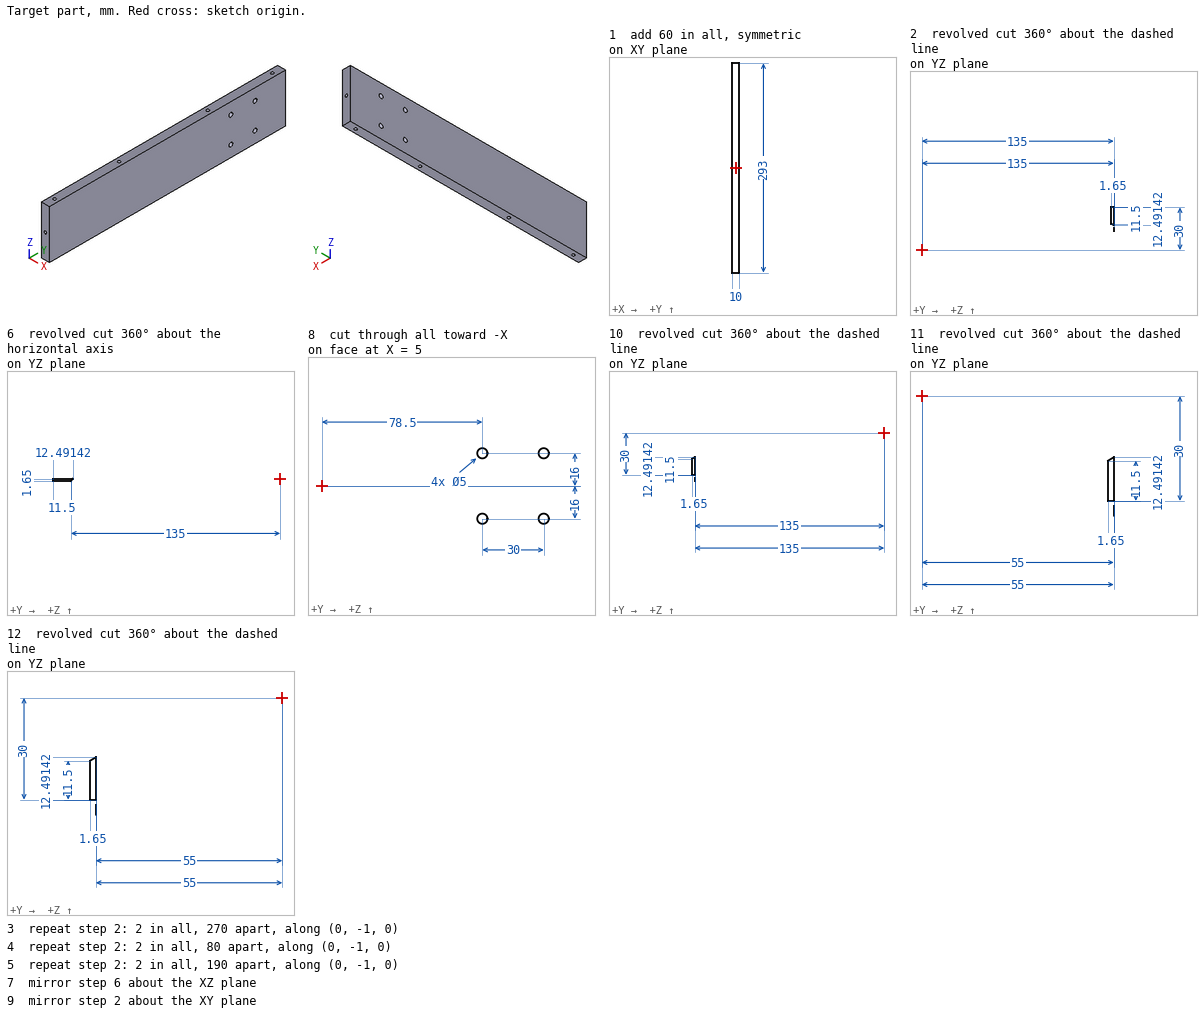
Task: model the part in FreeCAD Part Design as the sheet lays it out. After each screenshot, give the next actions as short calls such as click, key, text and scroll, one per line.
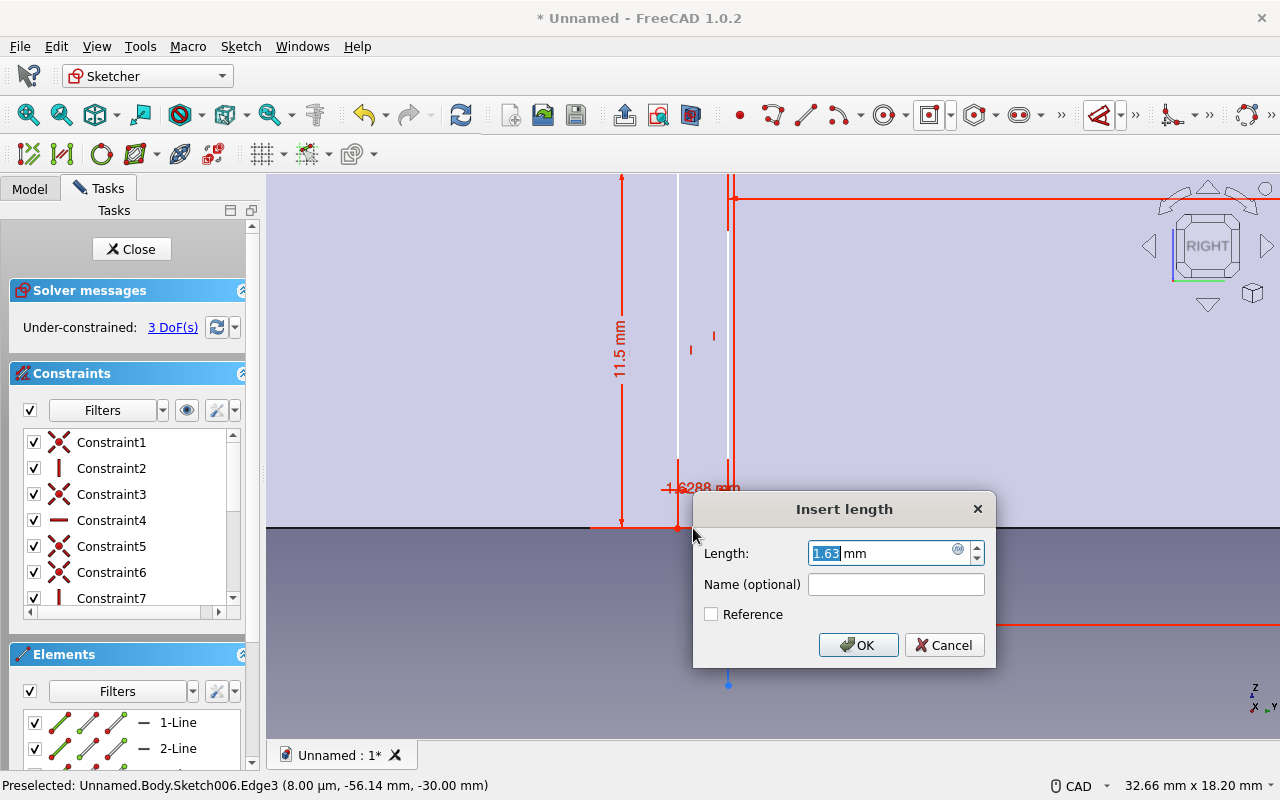
text(1.65)
key(Return)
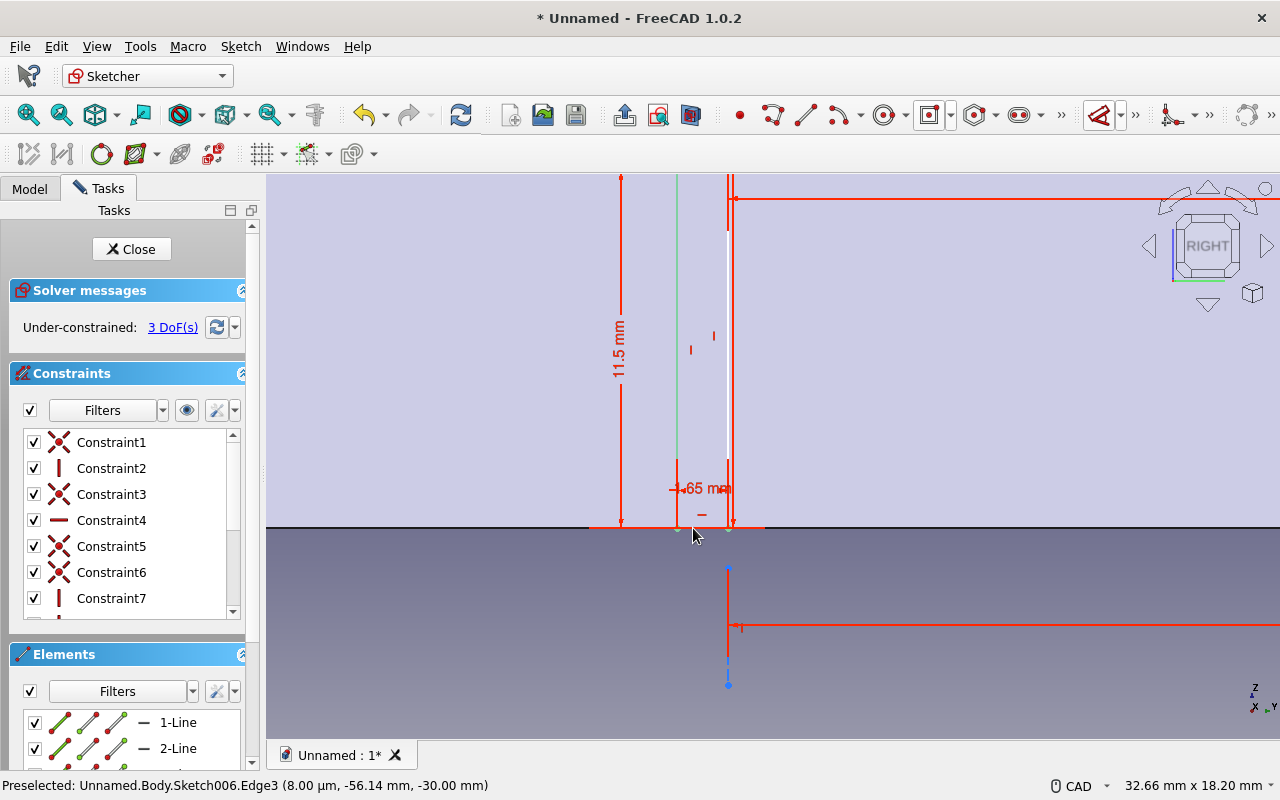
click(728, 412)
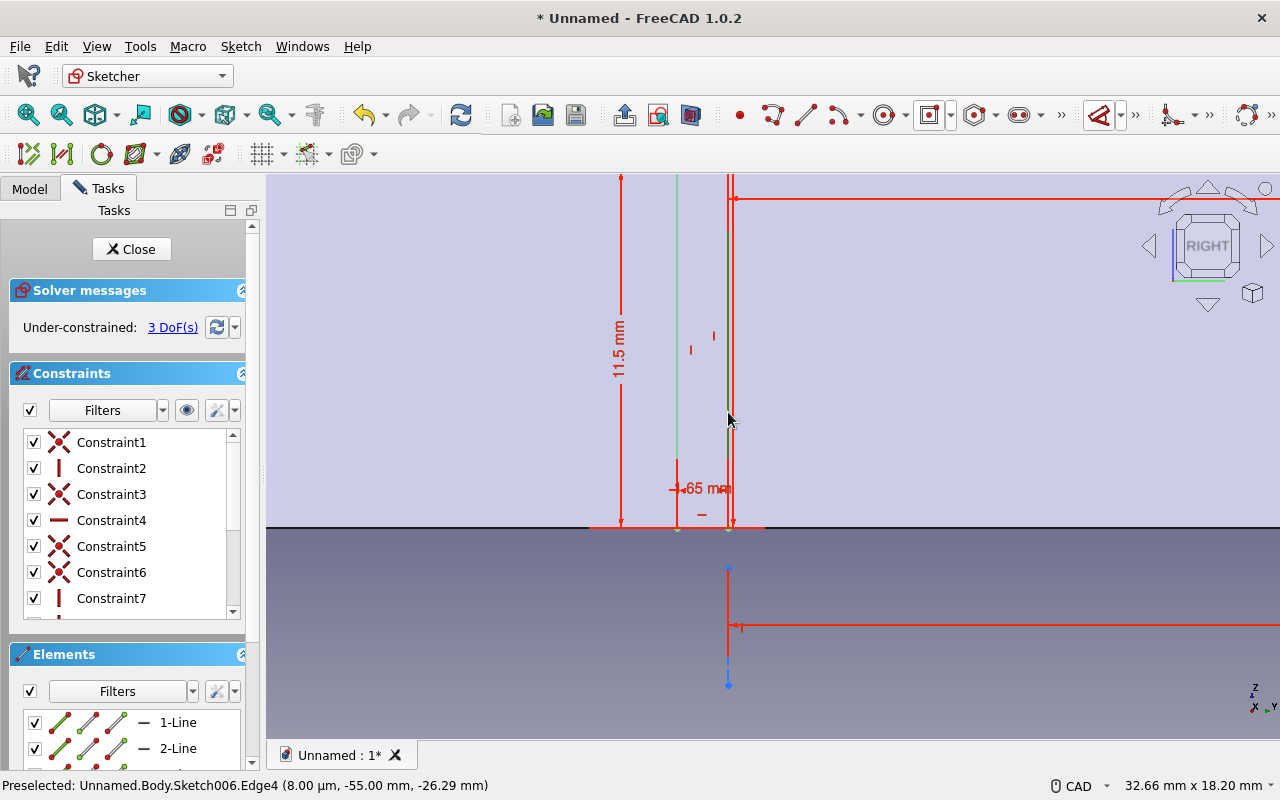
click(1120, 116)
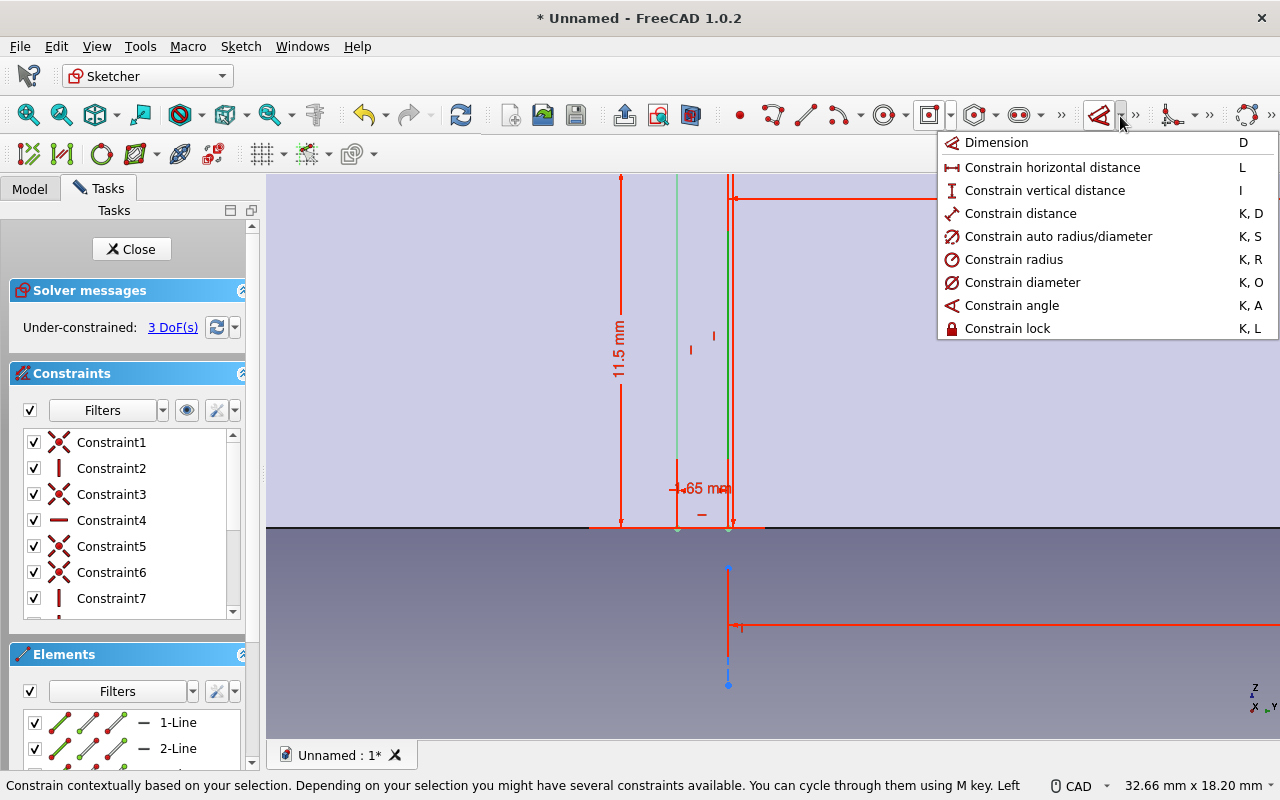
click(1108, 190)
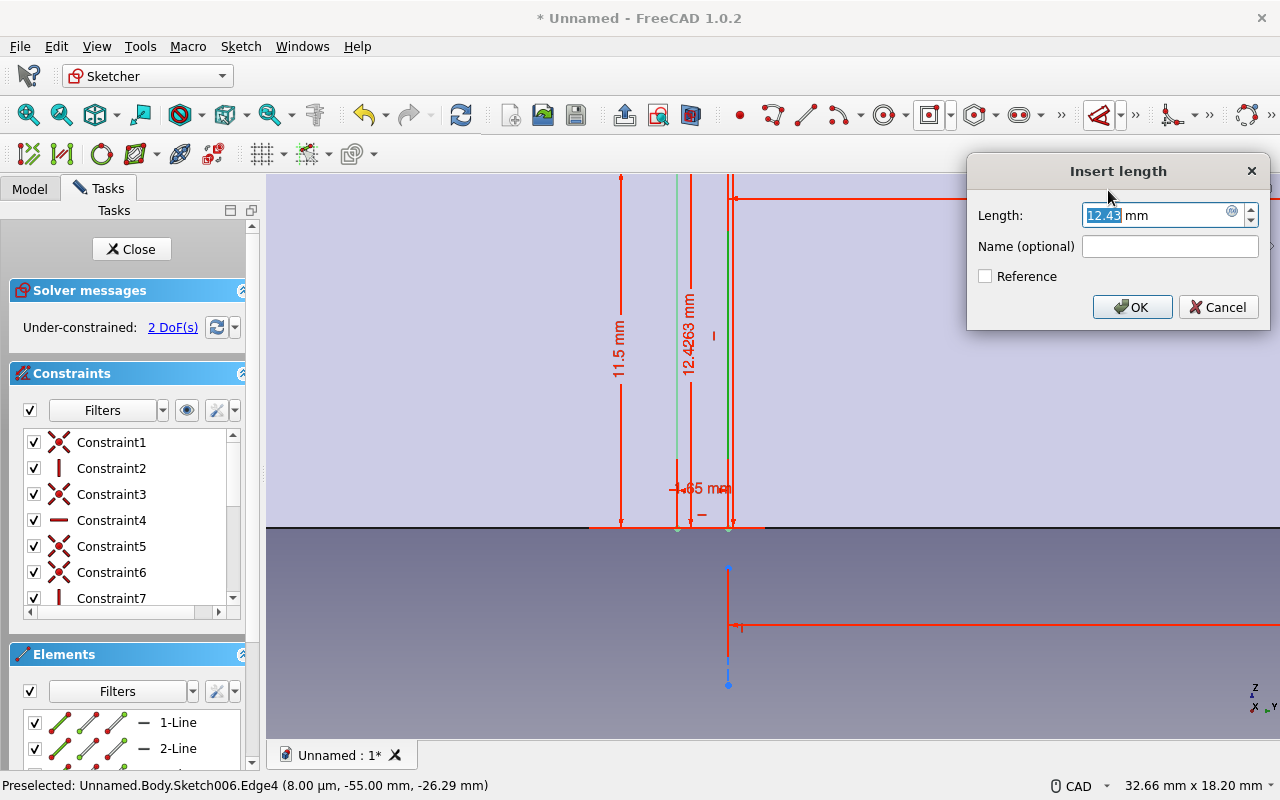
text(12.49142)
key(Return)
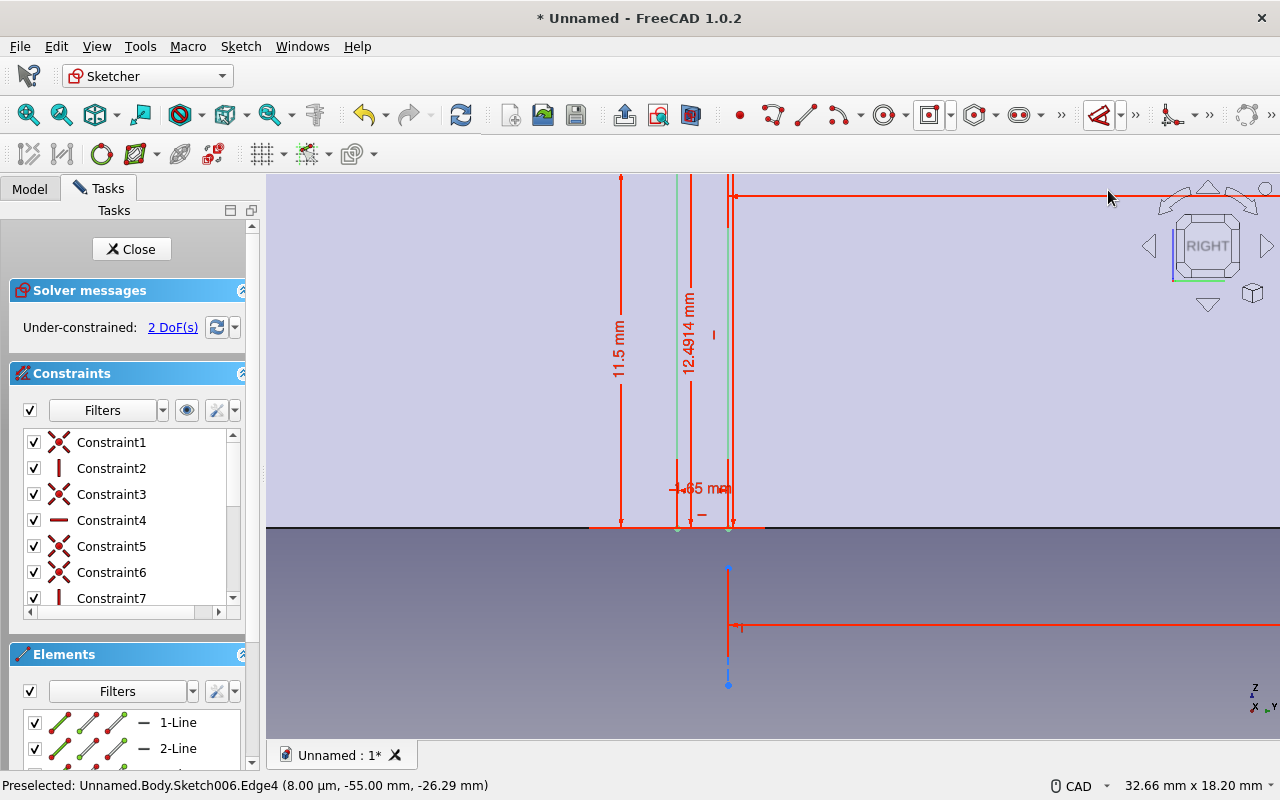
click(132, 249)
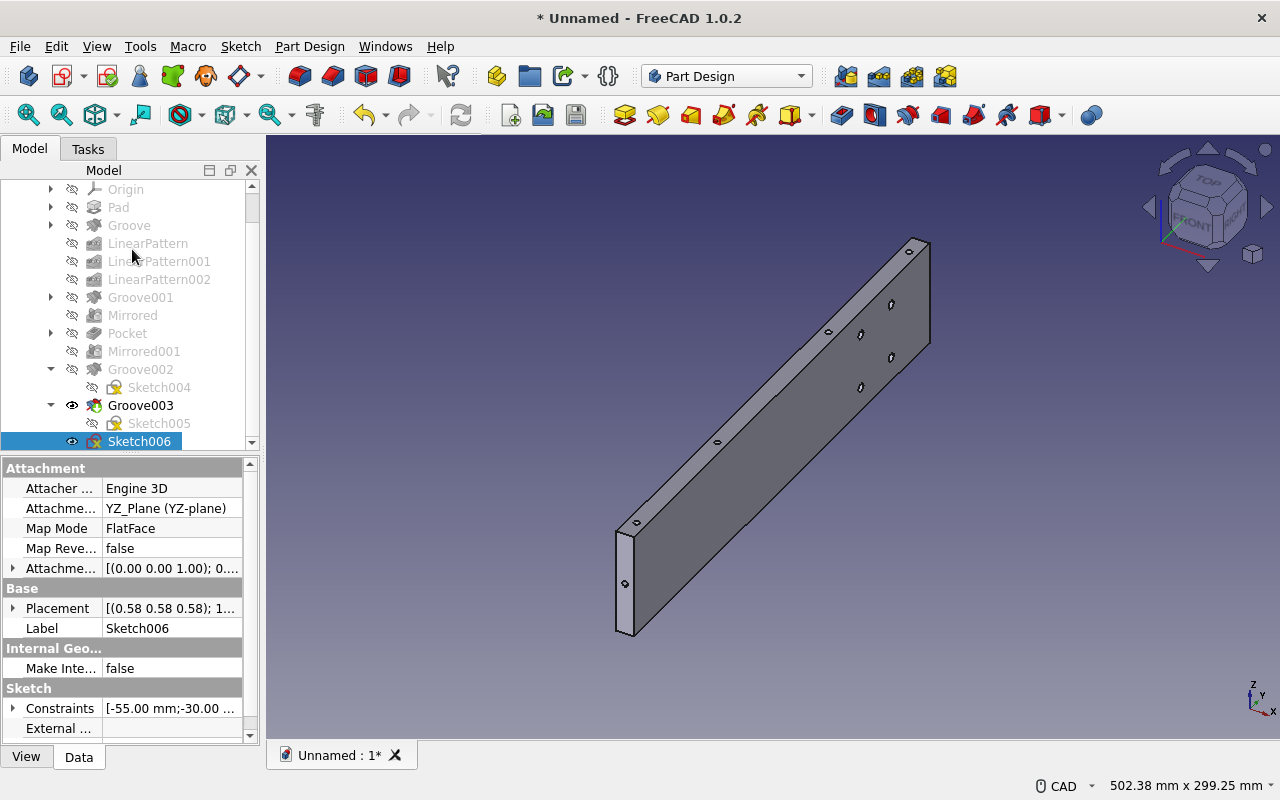
click(908, 116)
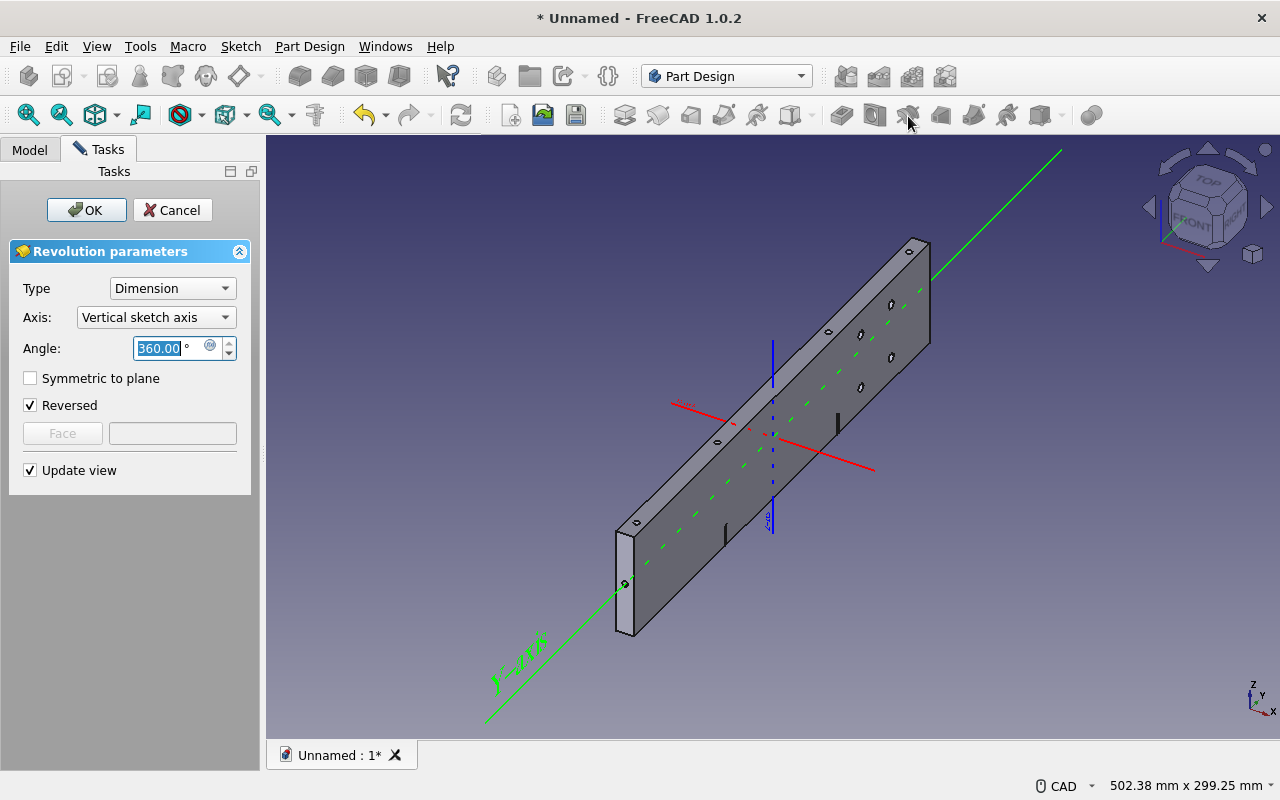
click(157, 318)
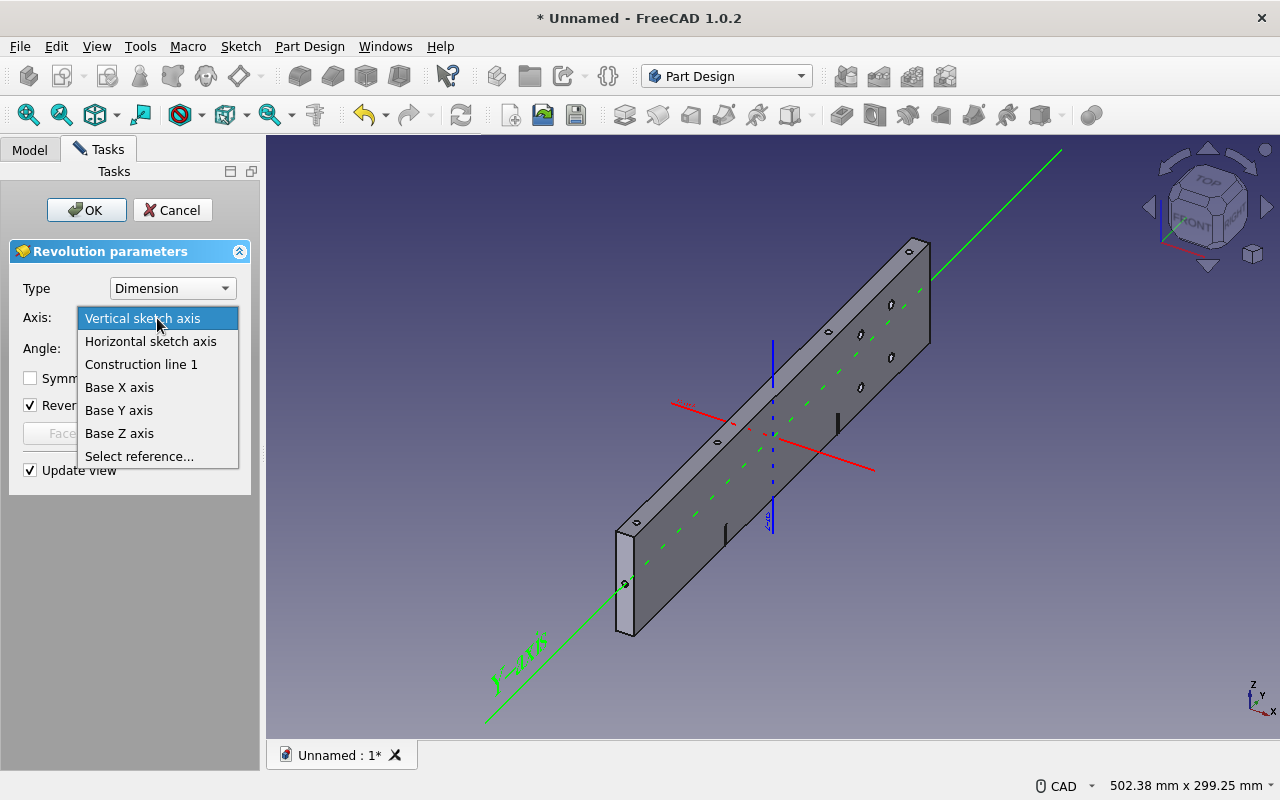
click(156, 364)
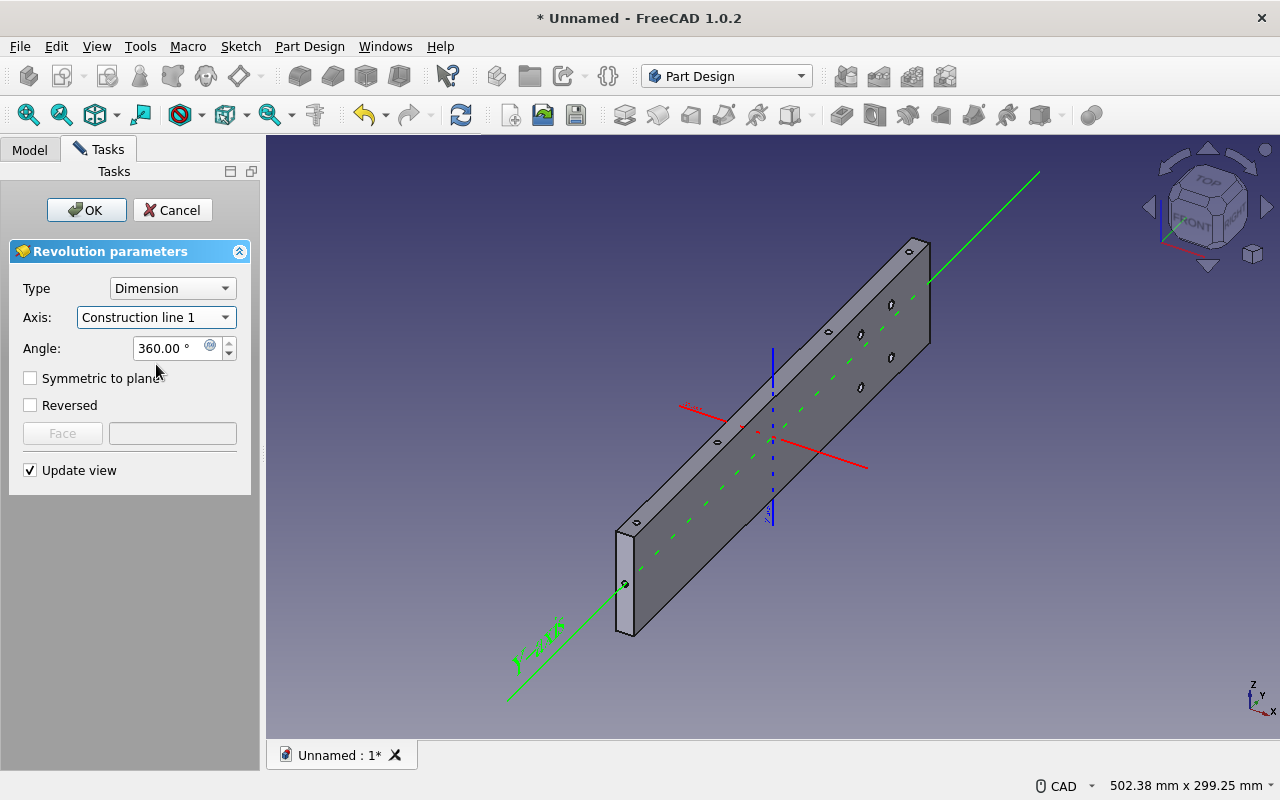
click(87, 210)